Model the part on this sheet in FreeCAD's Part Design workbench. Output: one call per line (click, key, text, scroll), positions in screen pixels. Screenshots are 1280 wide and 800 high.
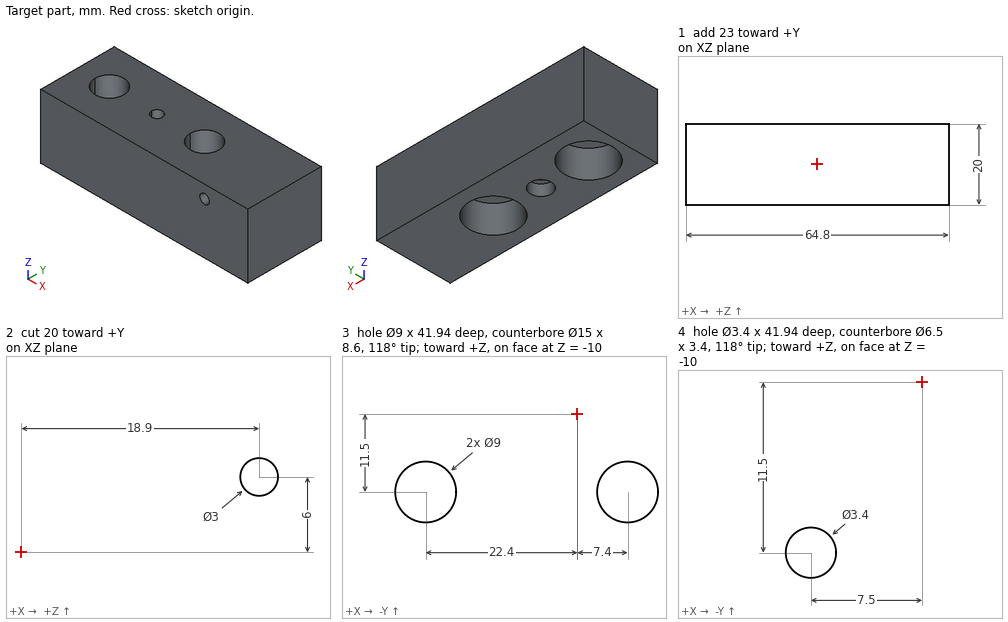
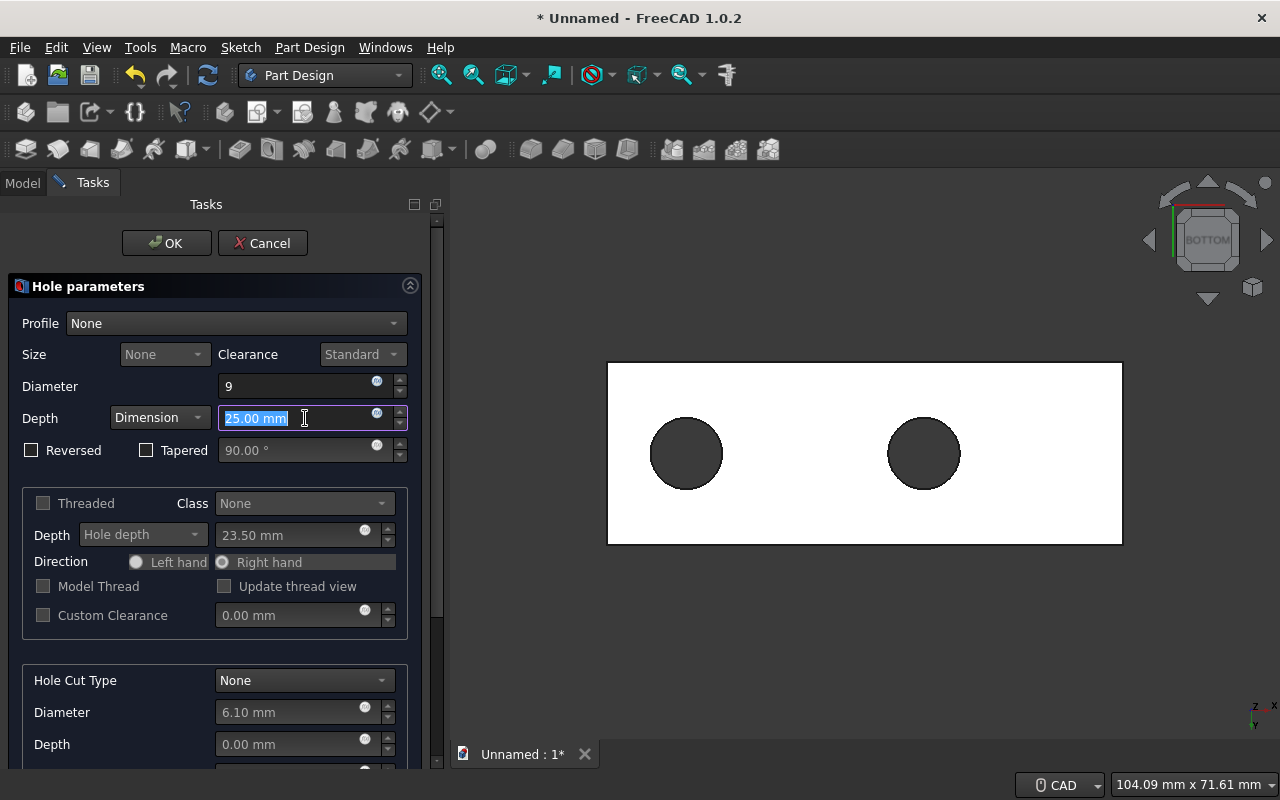
text(41.94)
key(Tab)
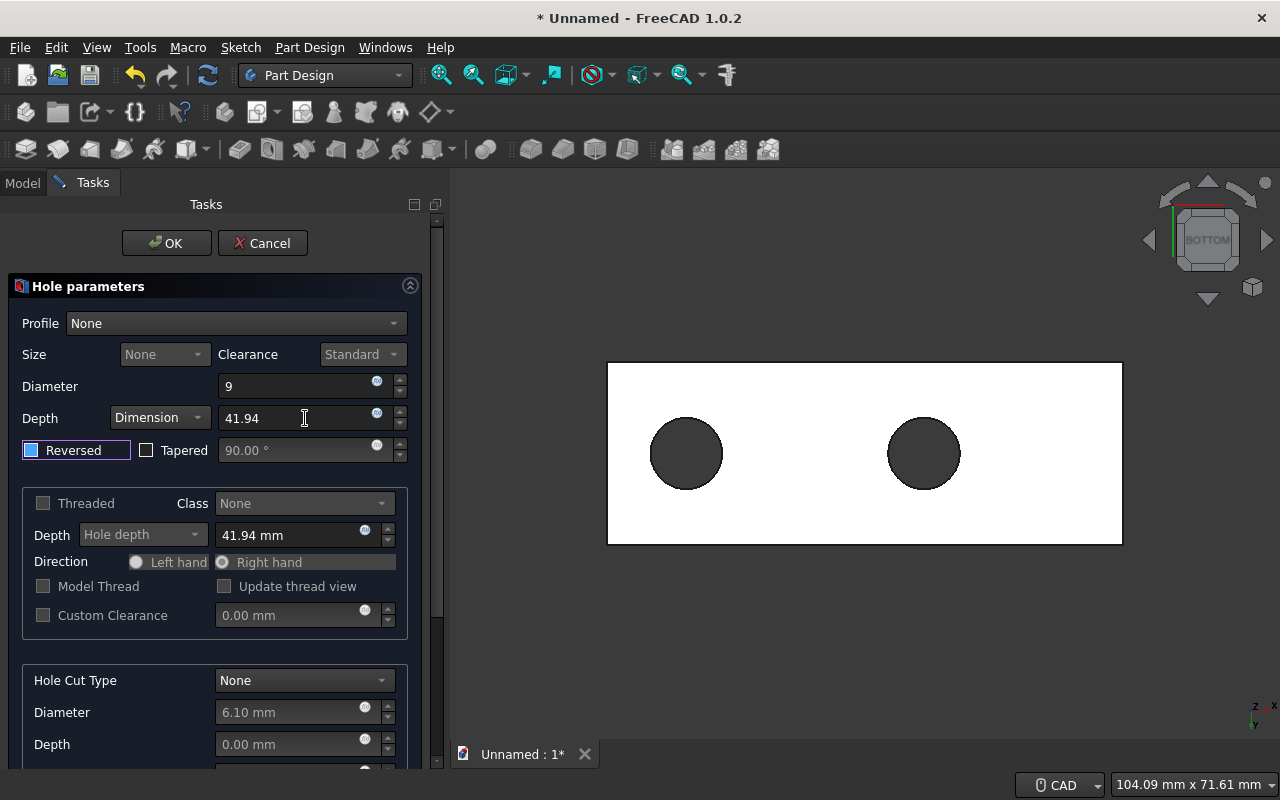
click(306, 680)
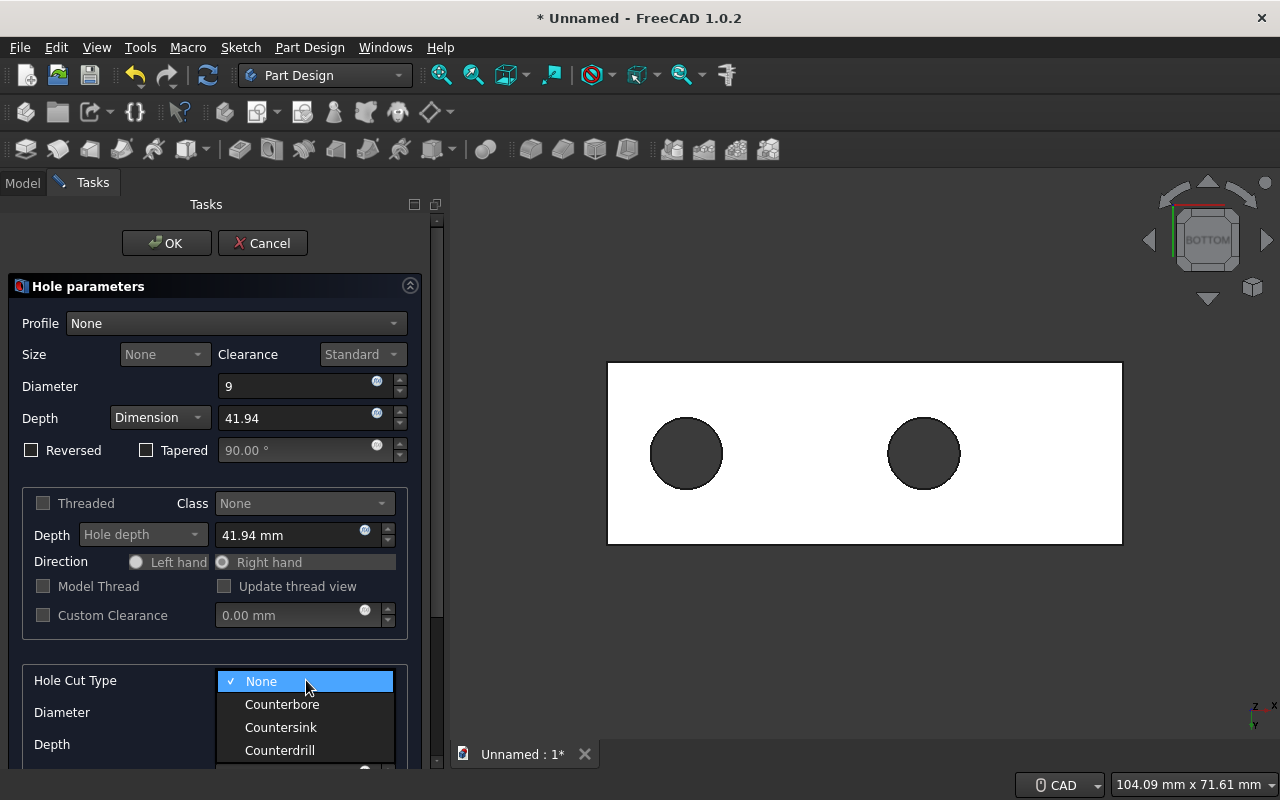
click(304, 704)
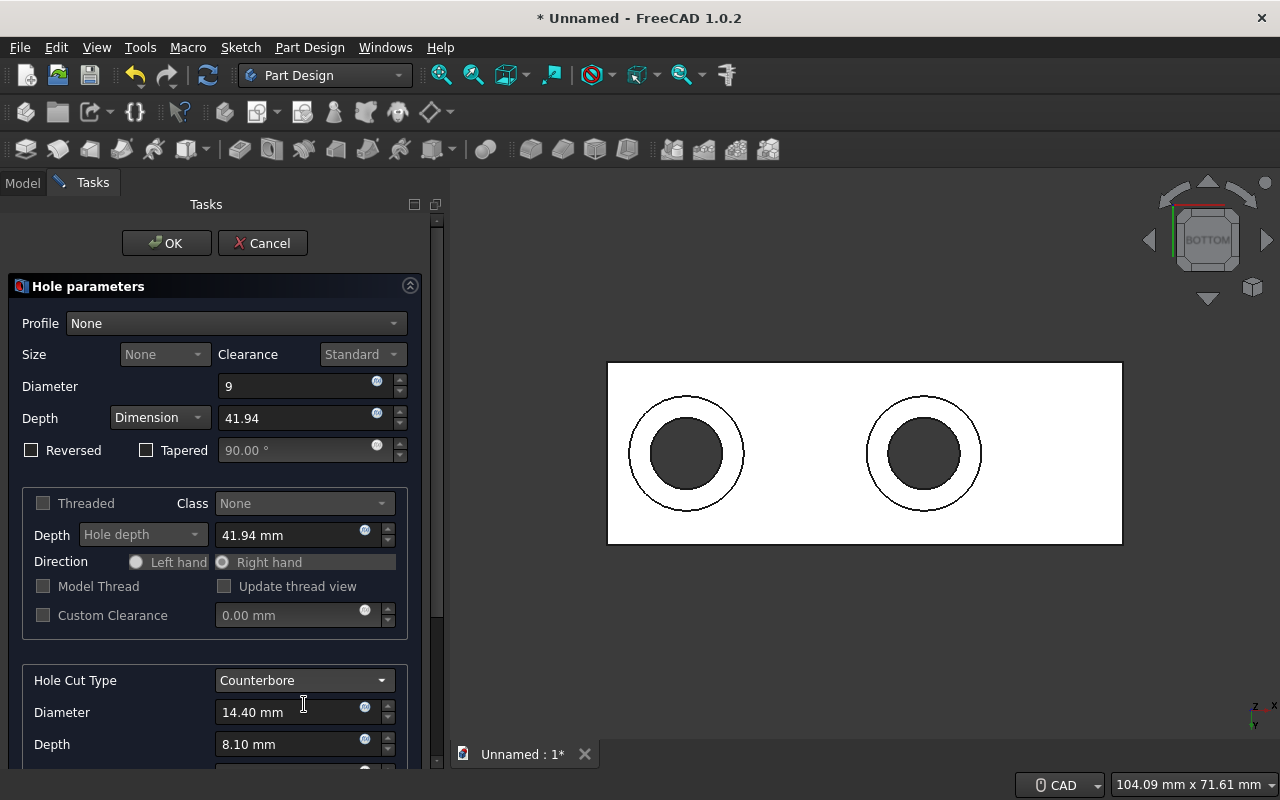
triple_click(298, 712)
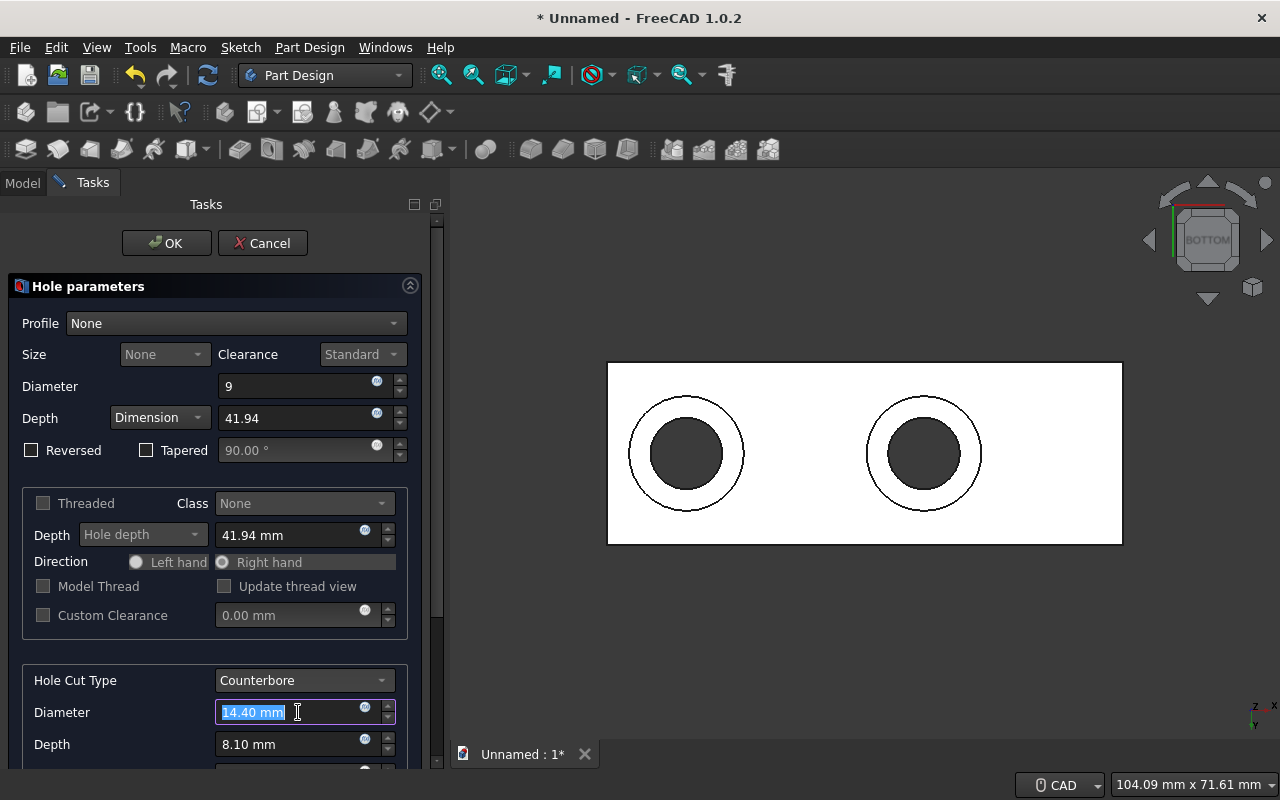
text(15)
key(Tab)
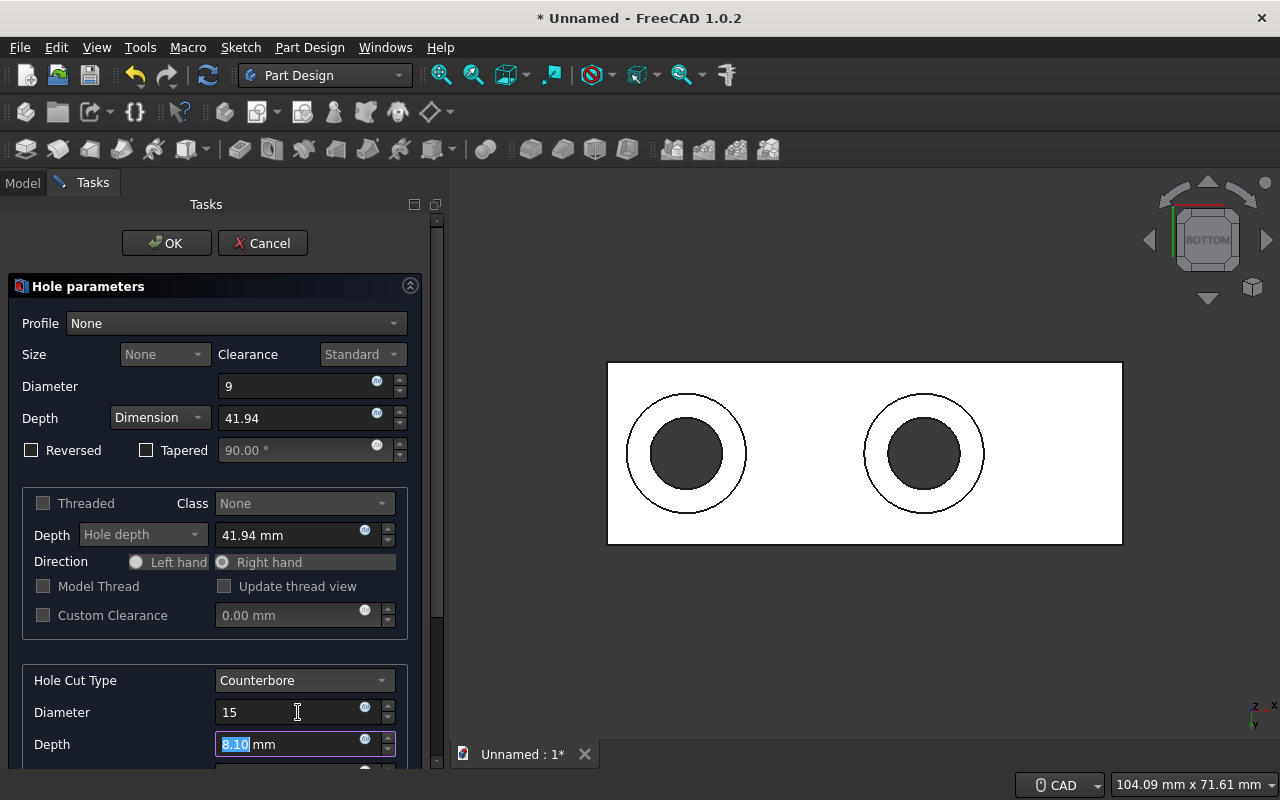
text(8.6)
key(Tab)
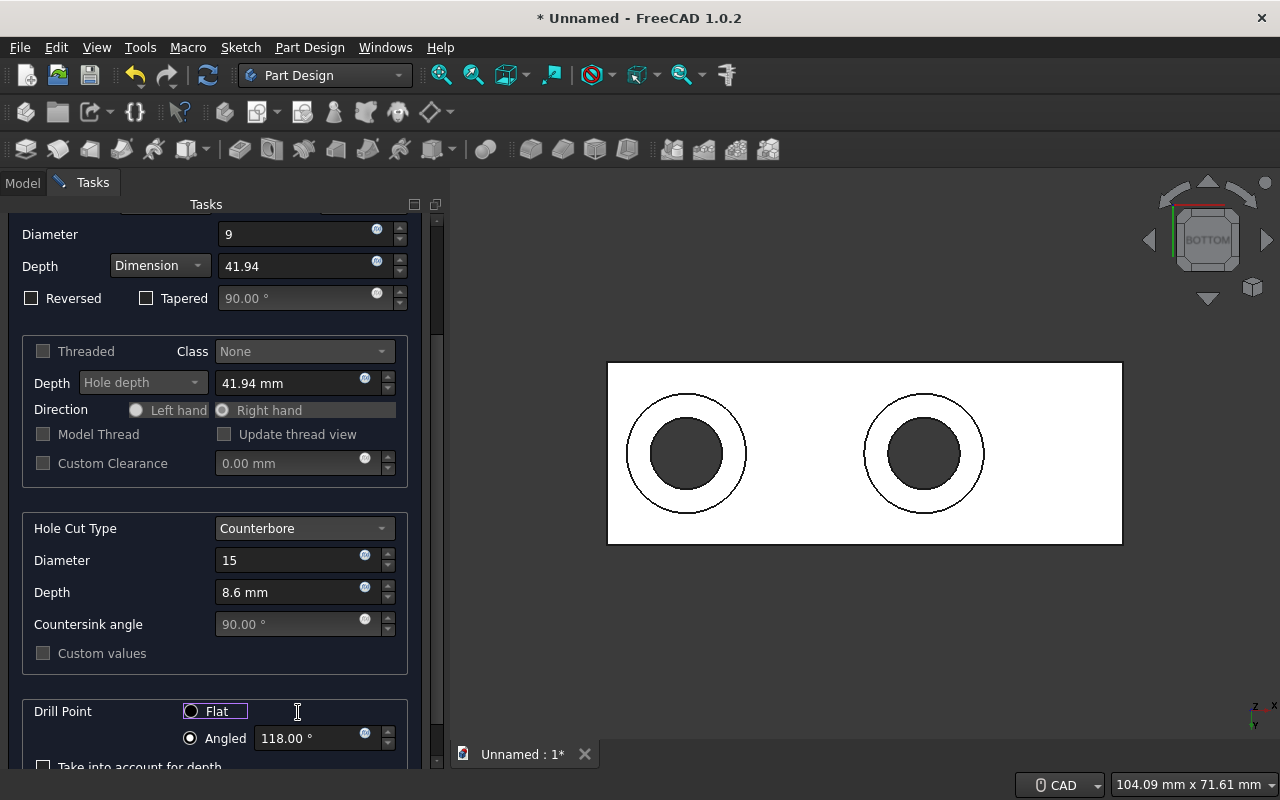
scroll(437, 491, up, 4)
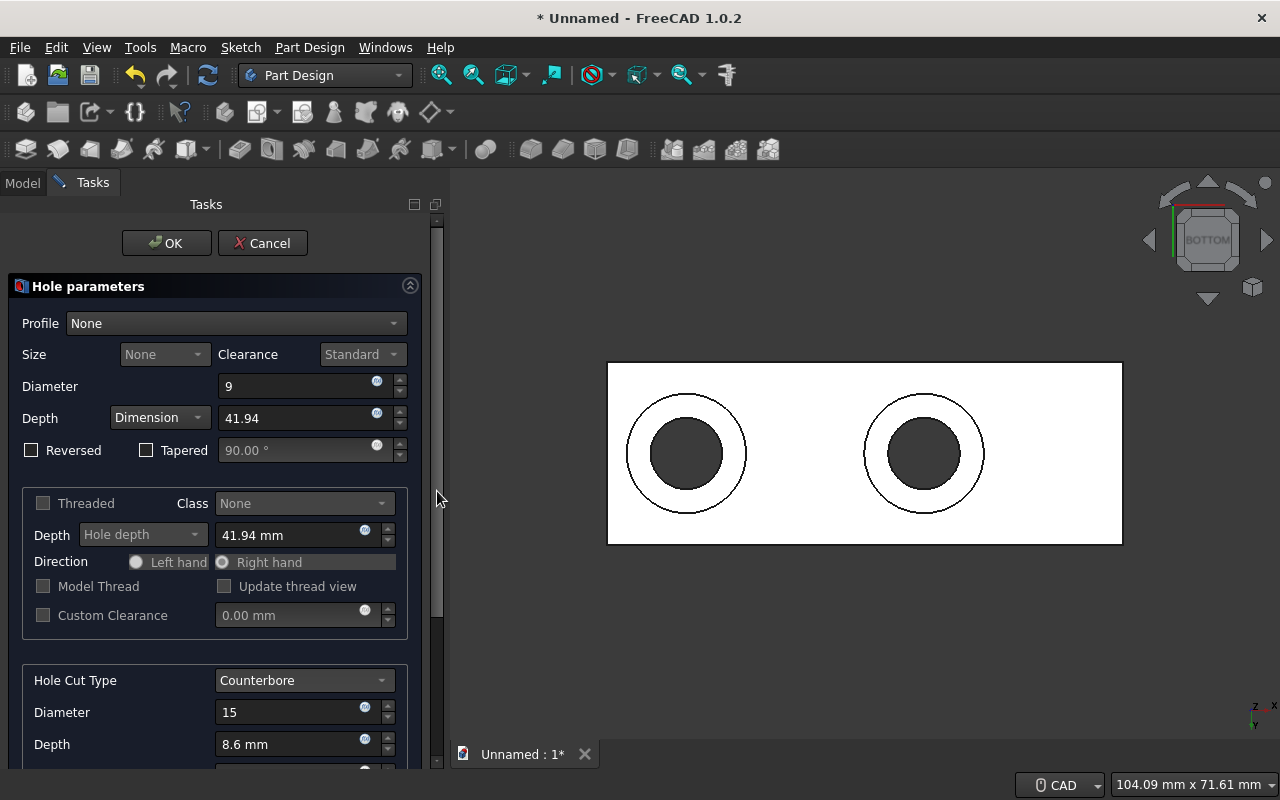
click(167, 243)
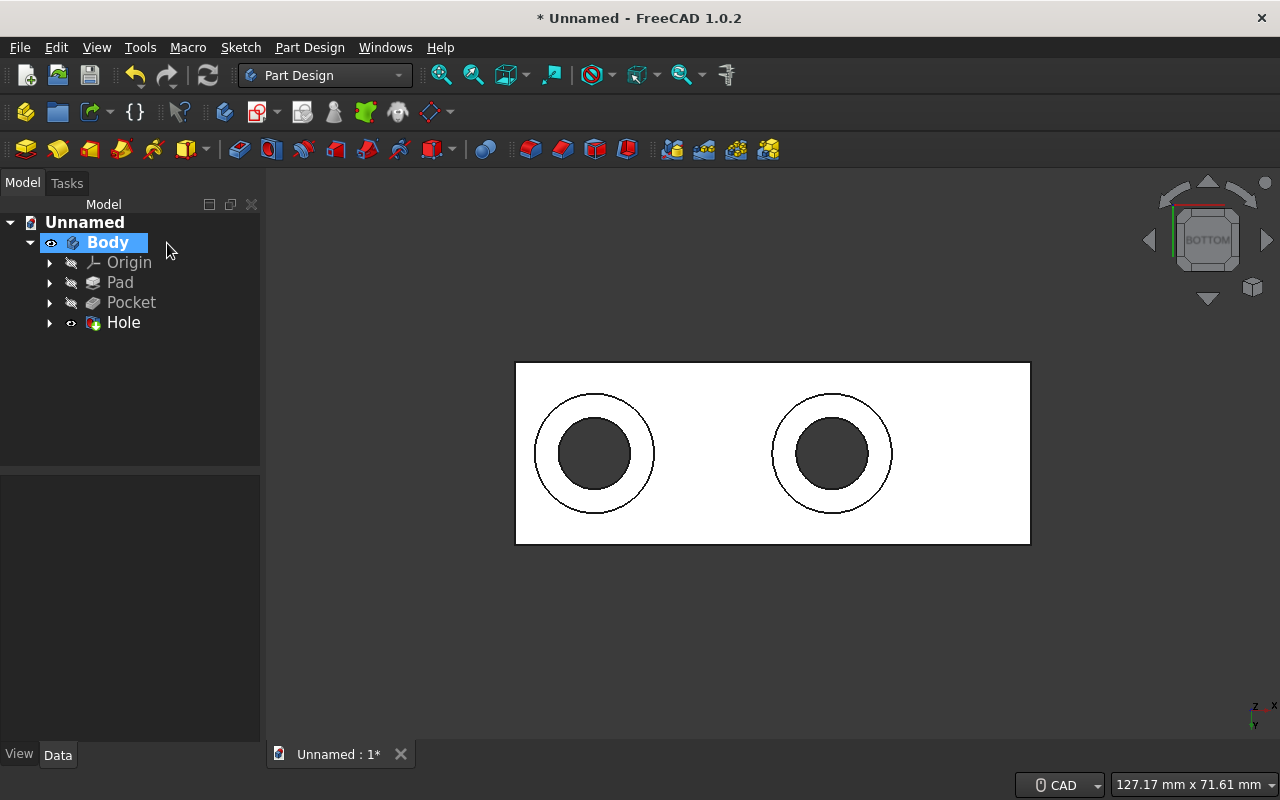
click(699, 479)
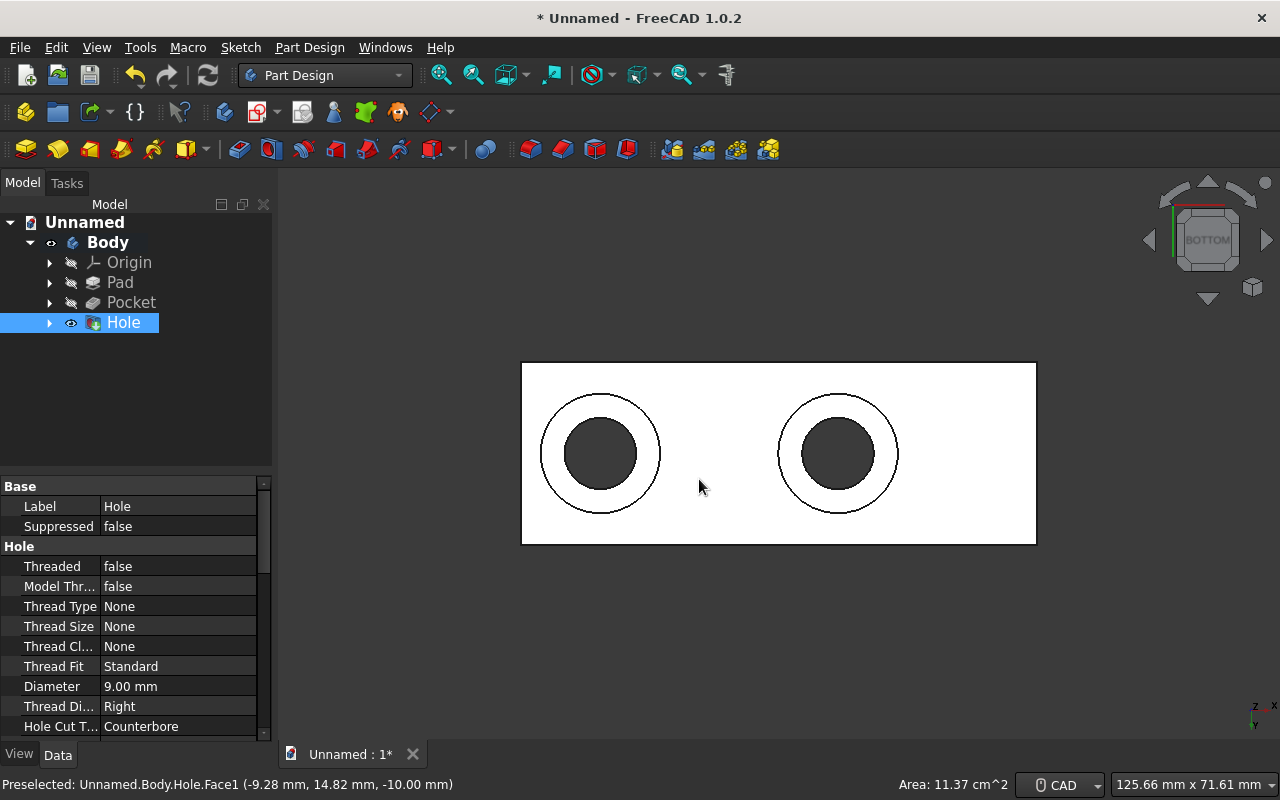
click(258, 112)